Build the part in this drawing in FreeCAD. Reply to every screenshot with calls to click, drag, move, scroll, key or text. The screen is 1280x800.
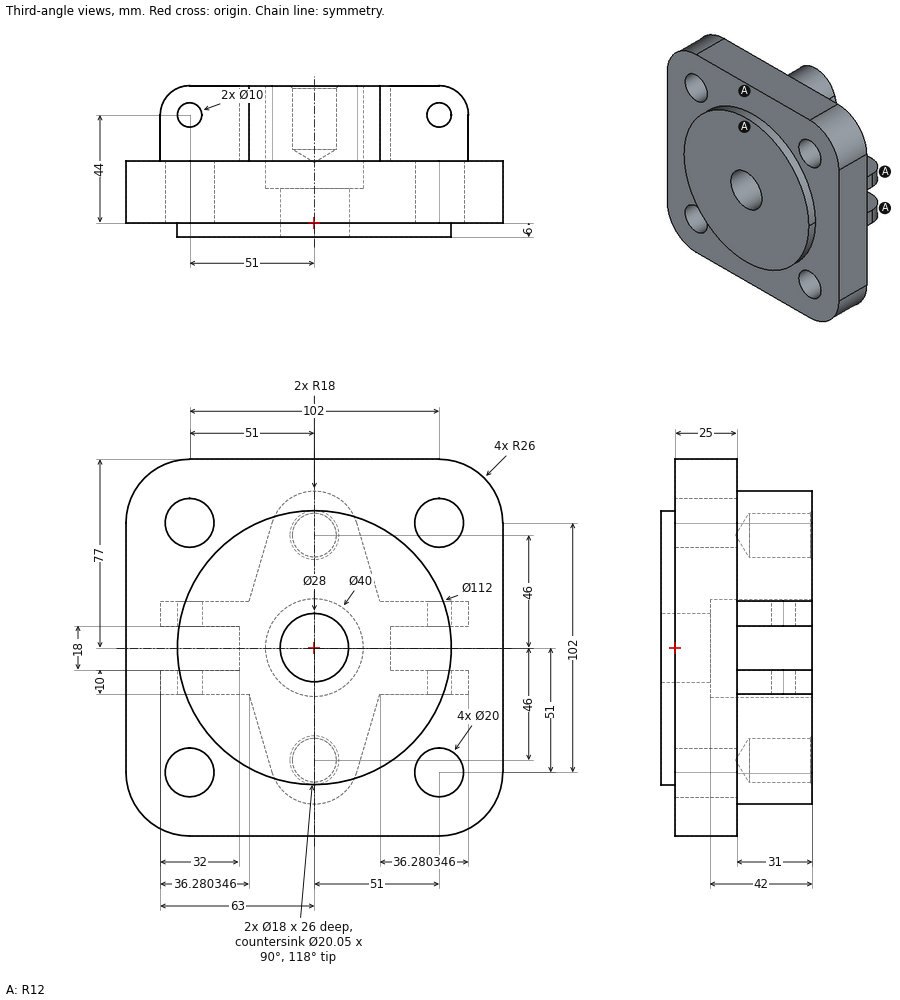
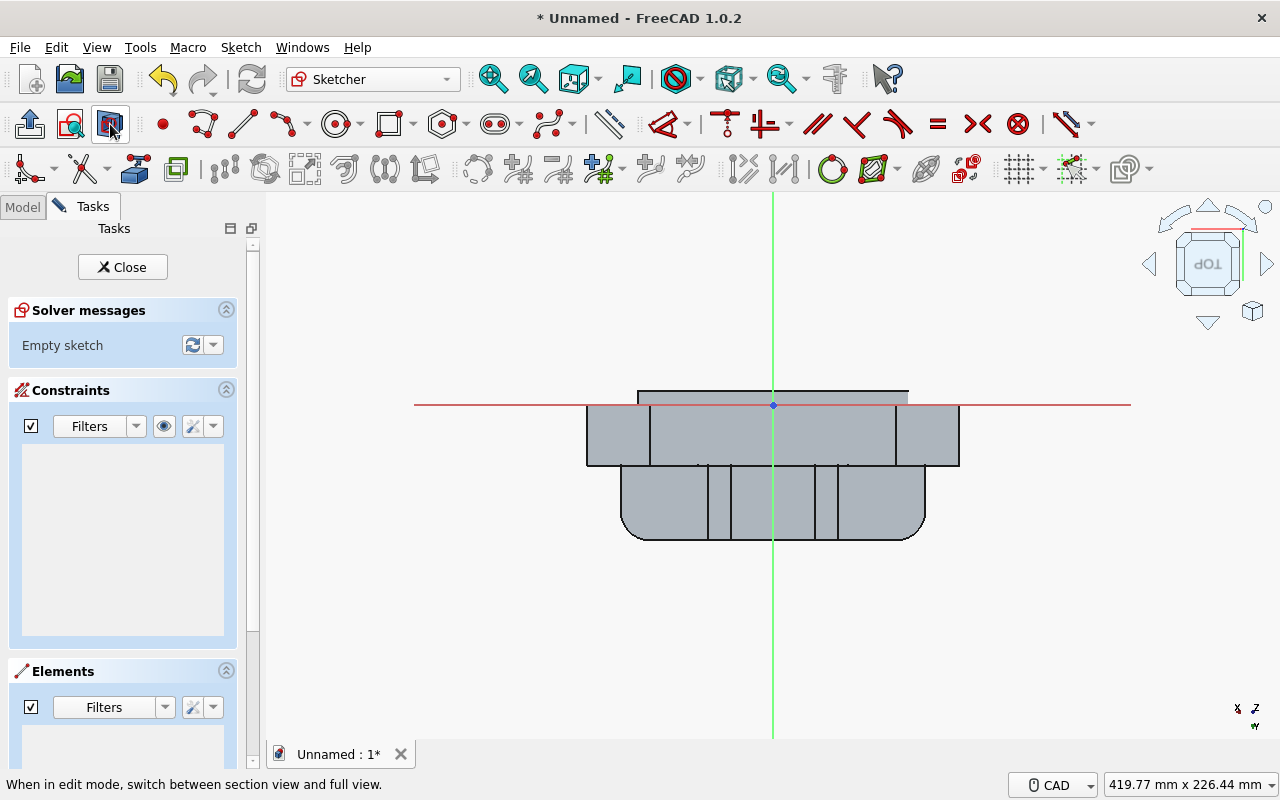
scroll(829, 463, up, 4)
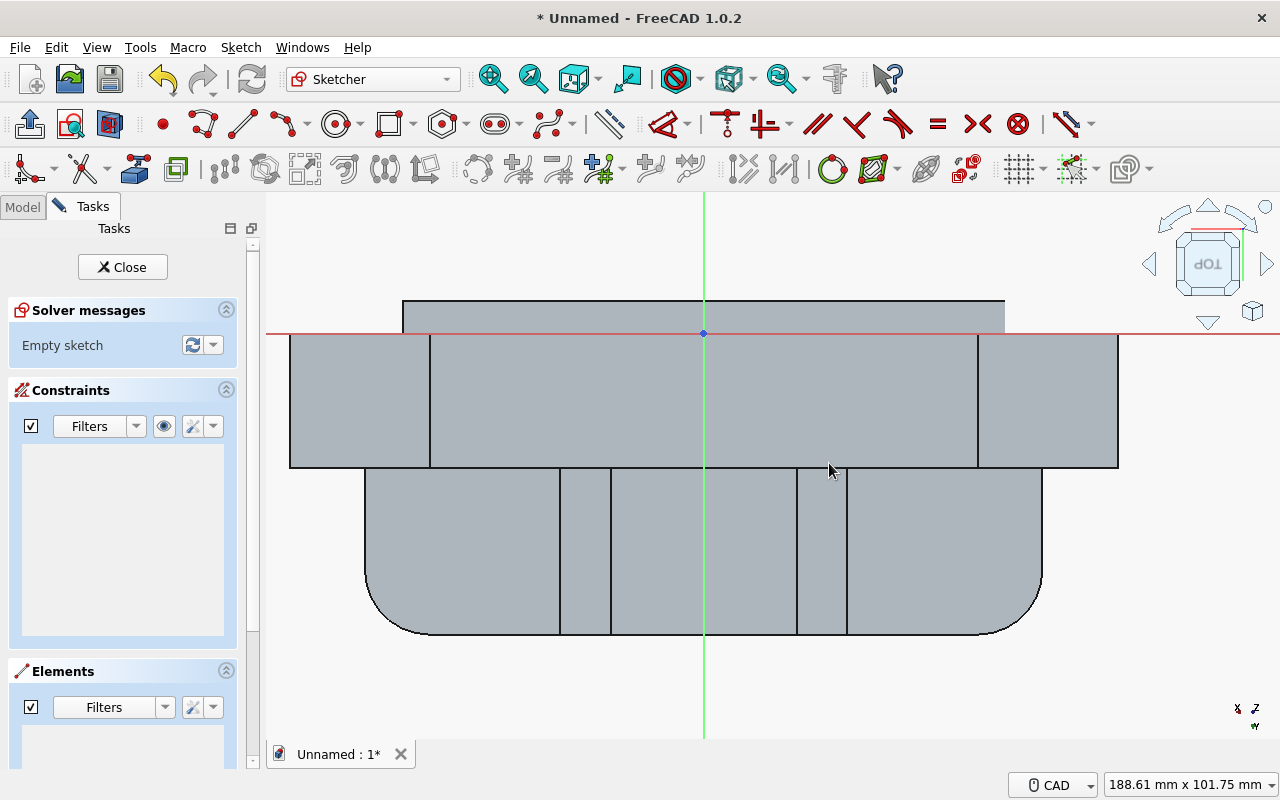
click(336, 124)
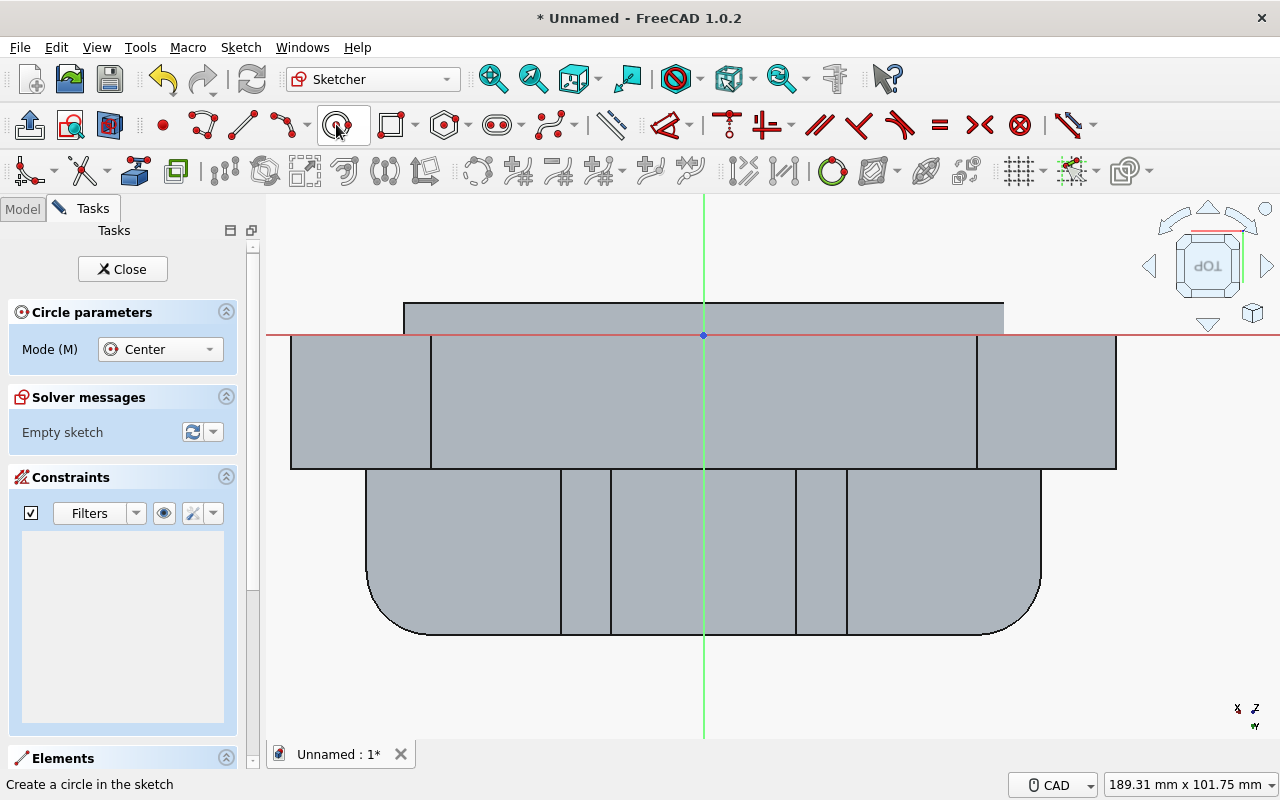
click(977, 571)
click(996, 552)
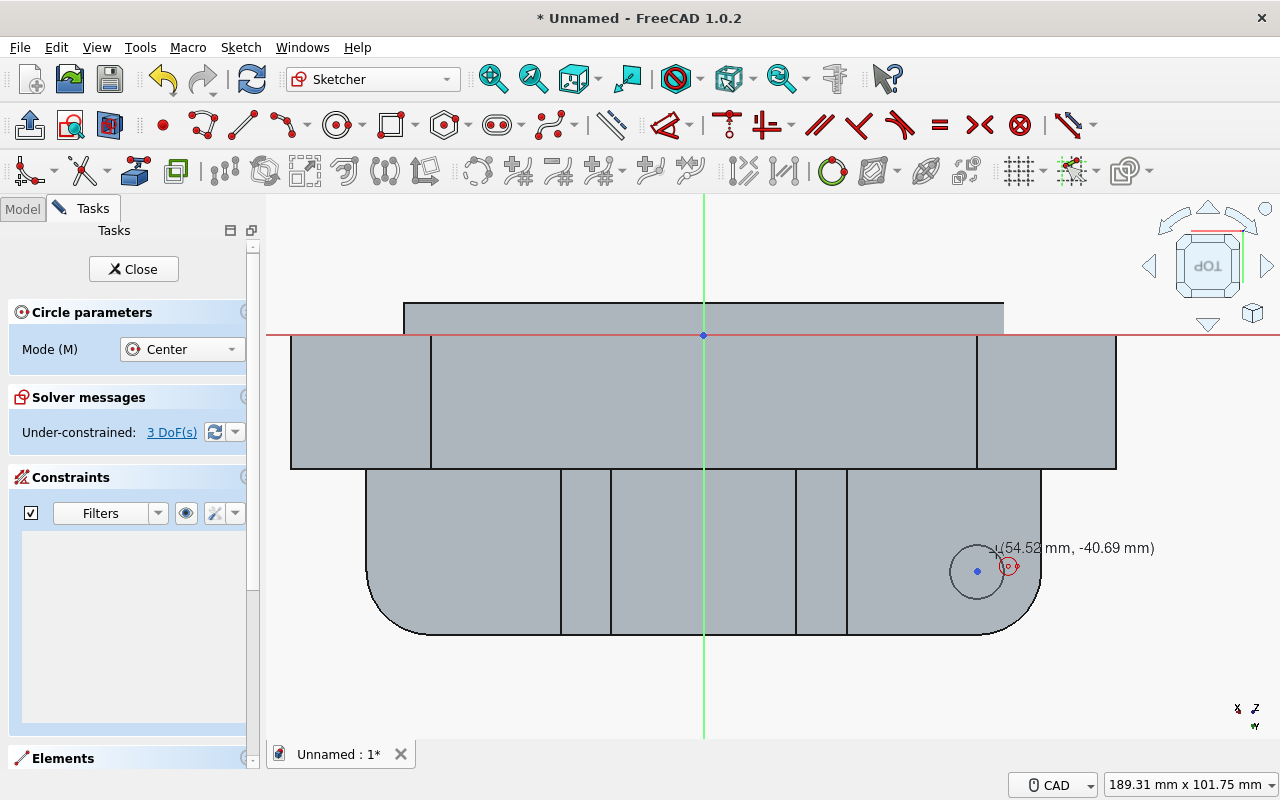
click(431, 571)
click(450, 552)
key(Escape)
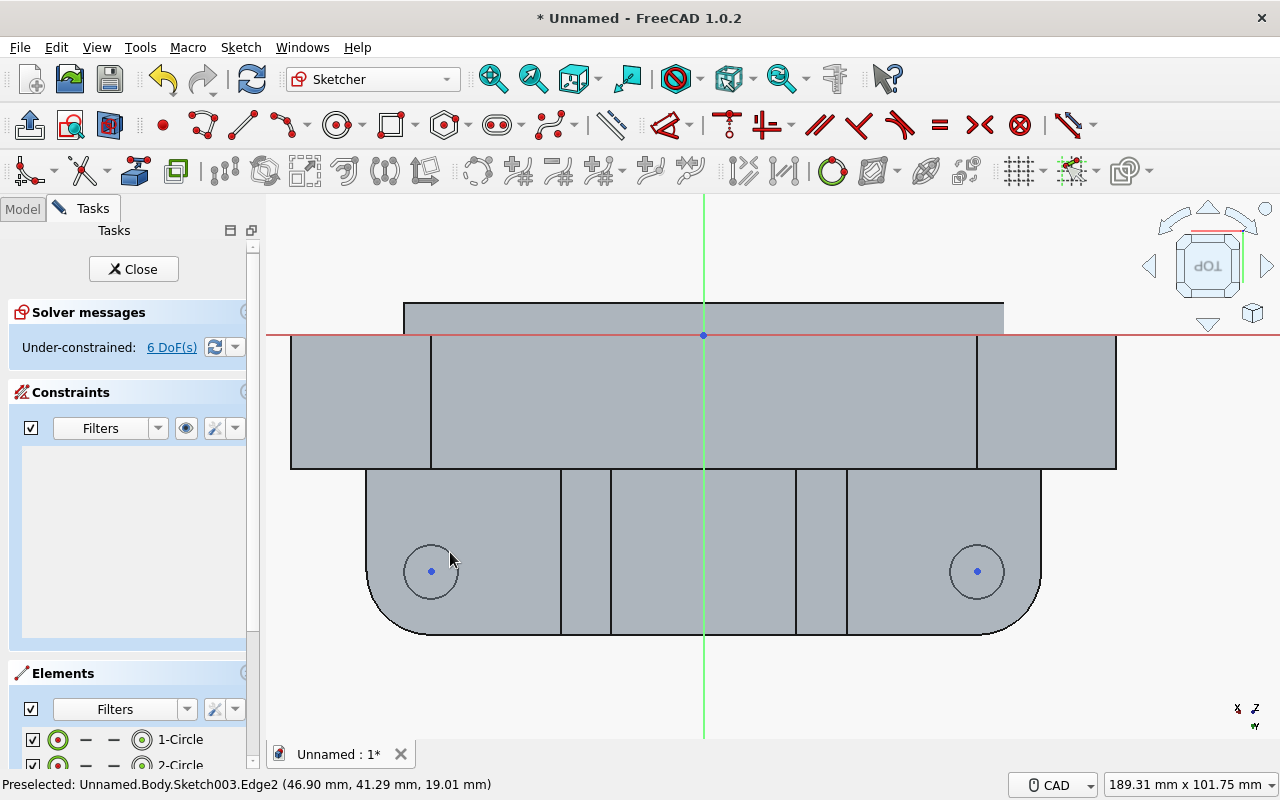
click(996, 553)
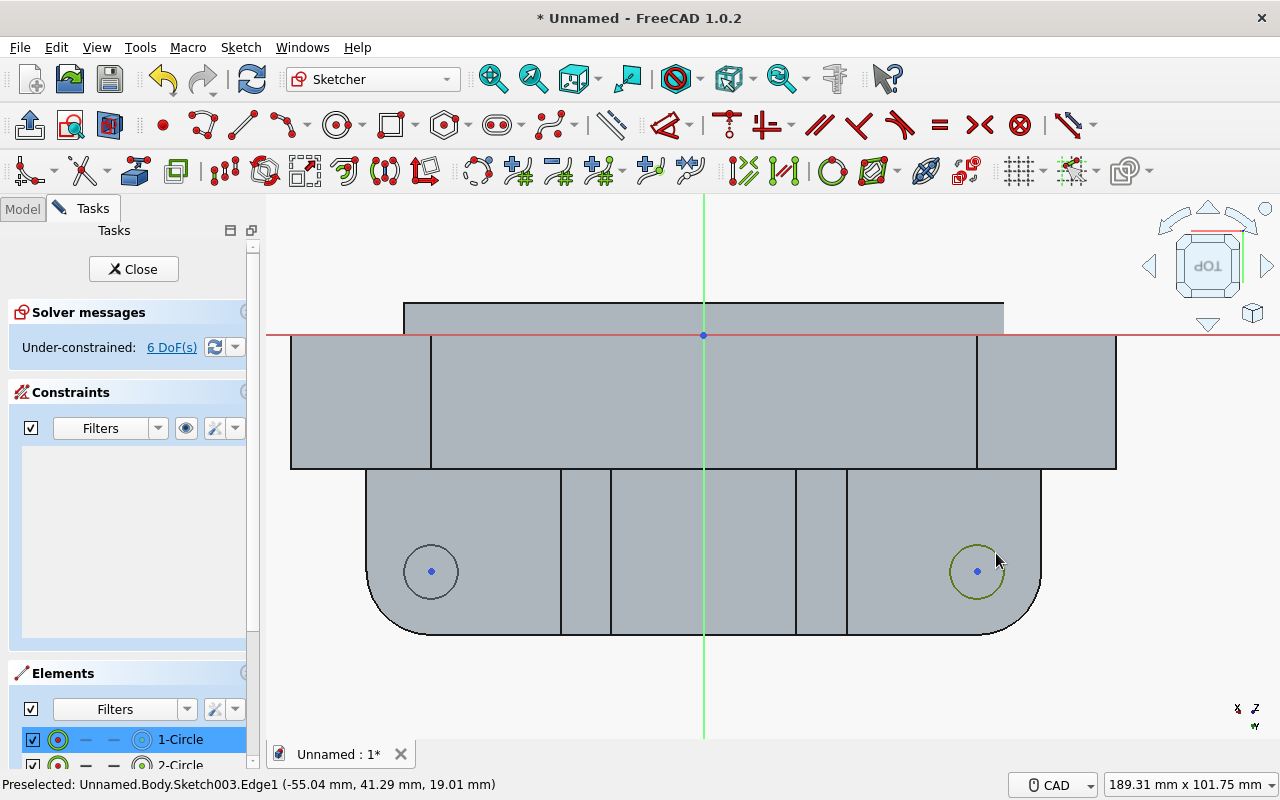
click(450, 553)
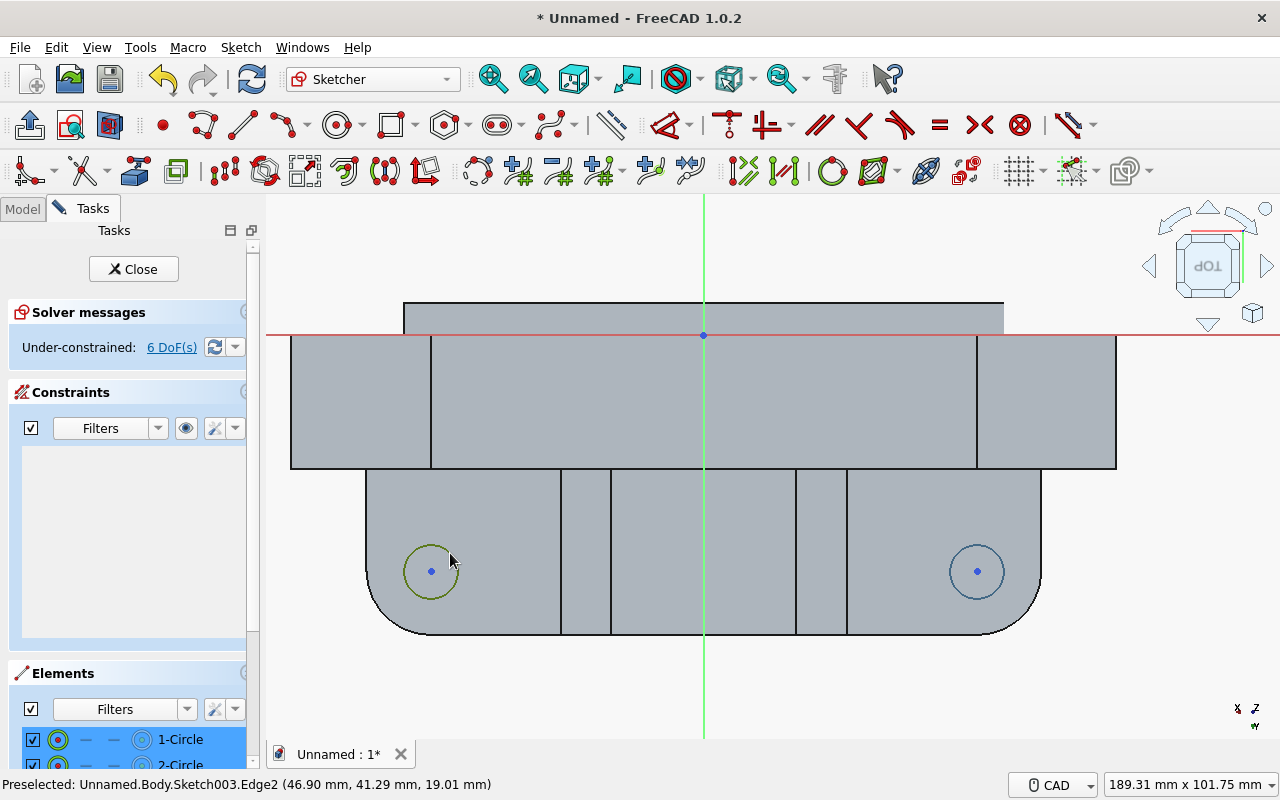
key(e)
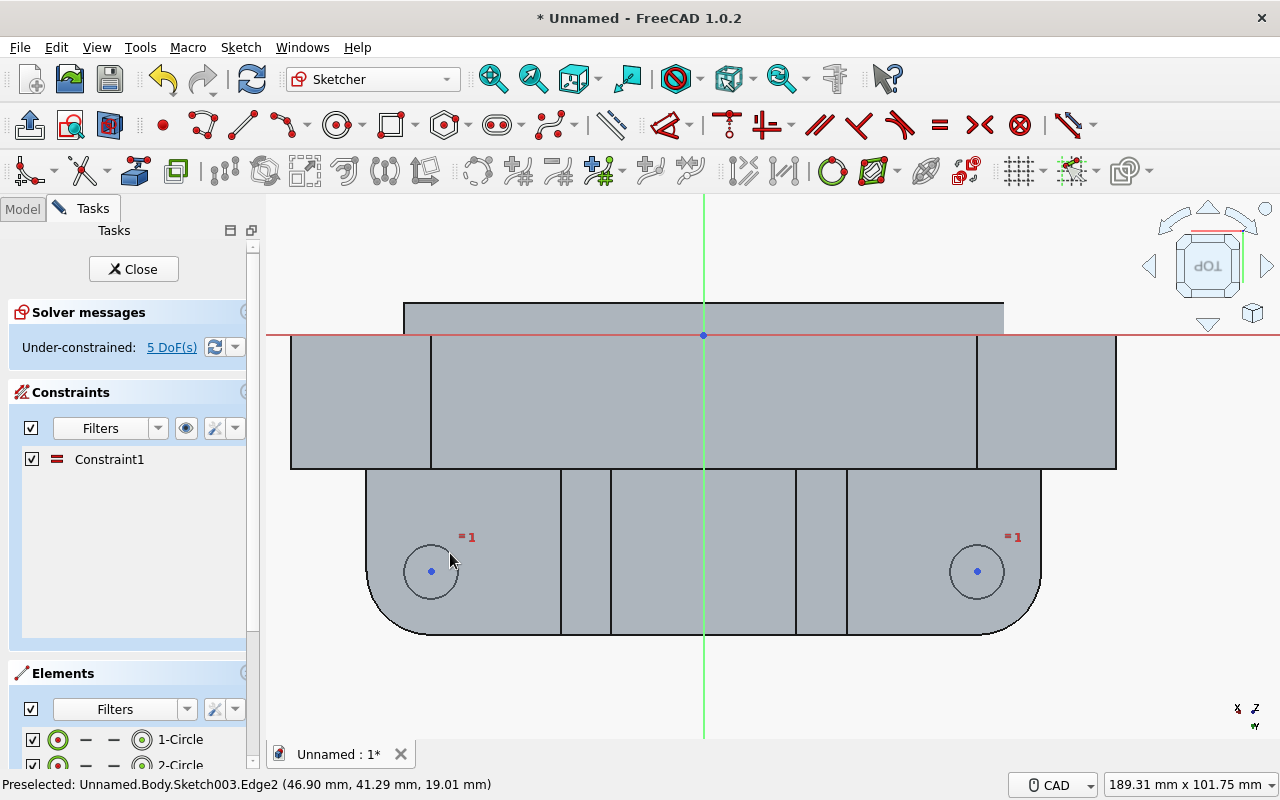
click(977, 572)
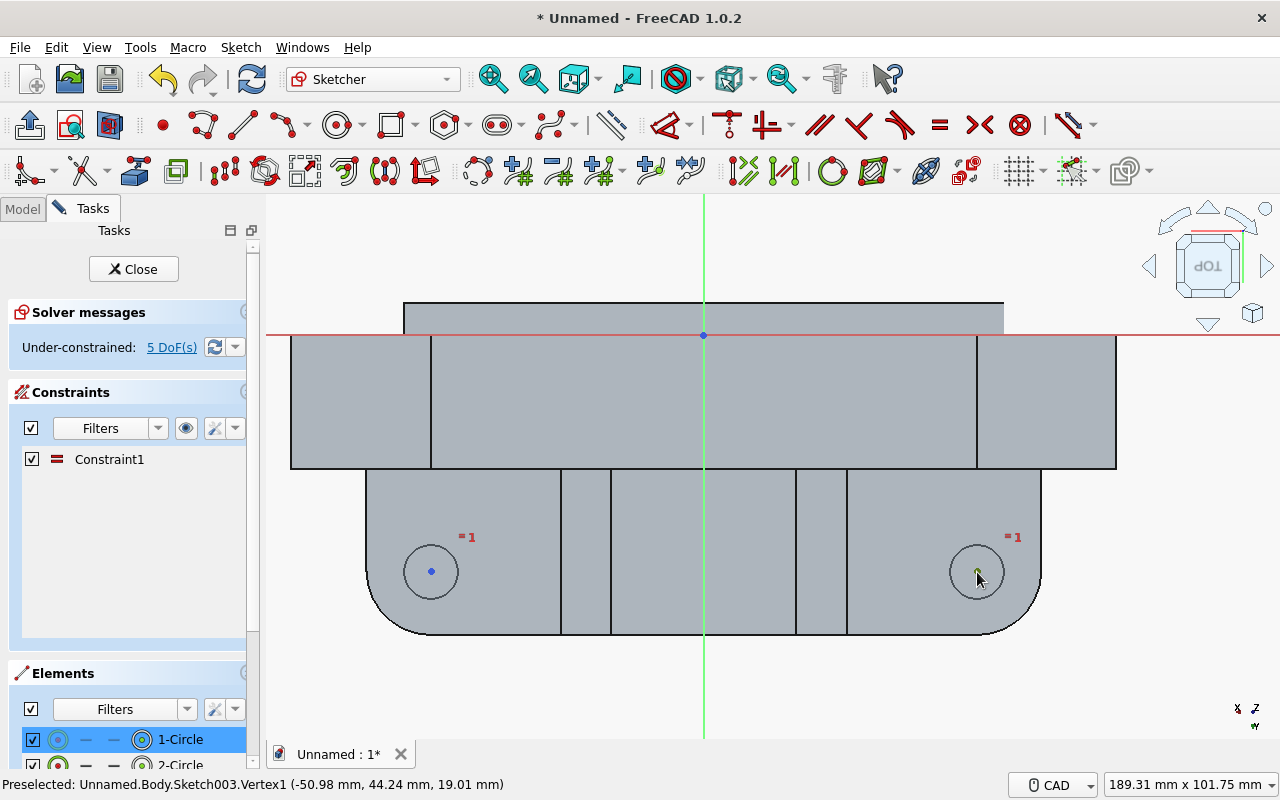
click(431, 572)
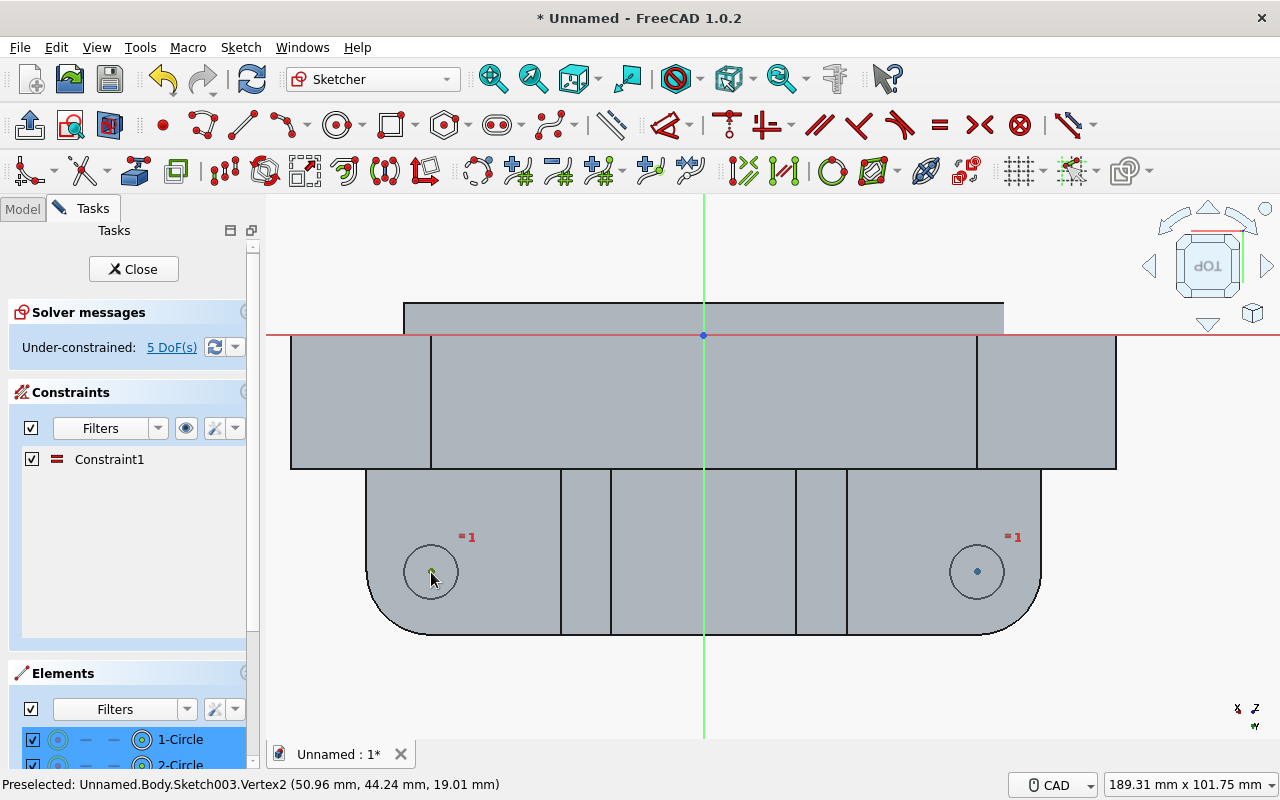
click(704, 676)